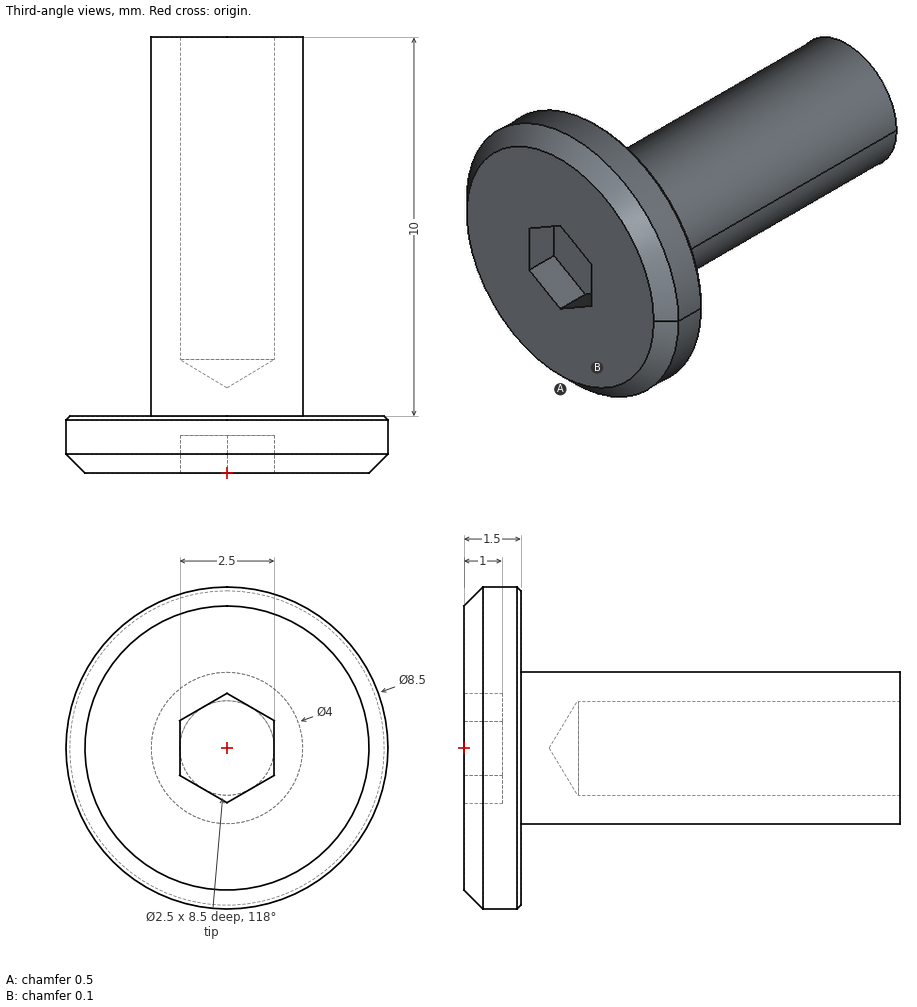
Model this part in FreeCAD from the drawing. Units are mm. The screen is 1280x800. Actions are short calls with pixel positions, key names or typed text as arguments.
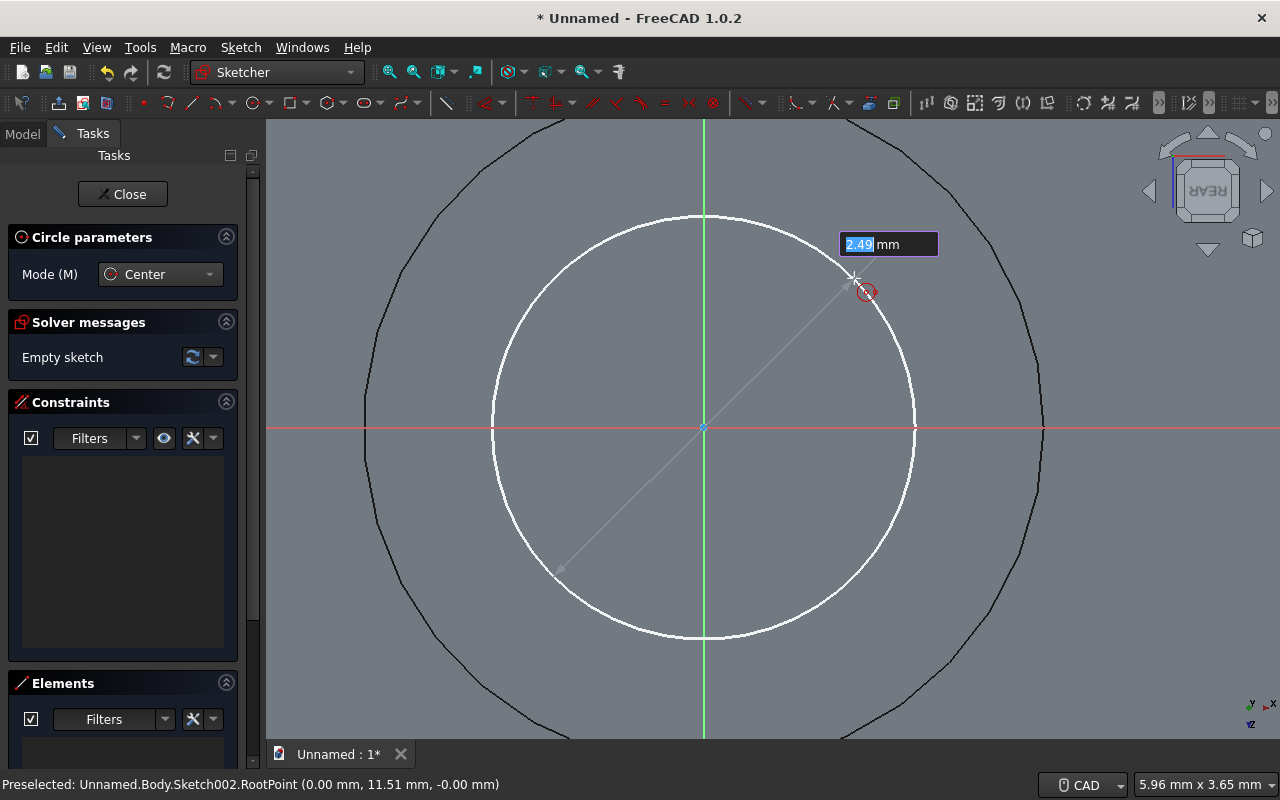
text(2.5)
key(Return)
key(Escape)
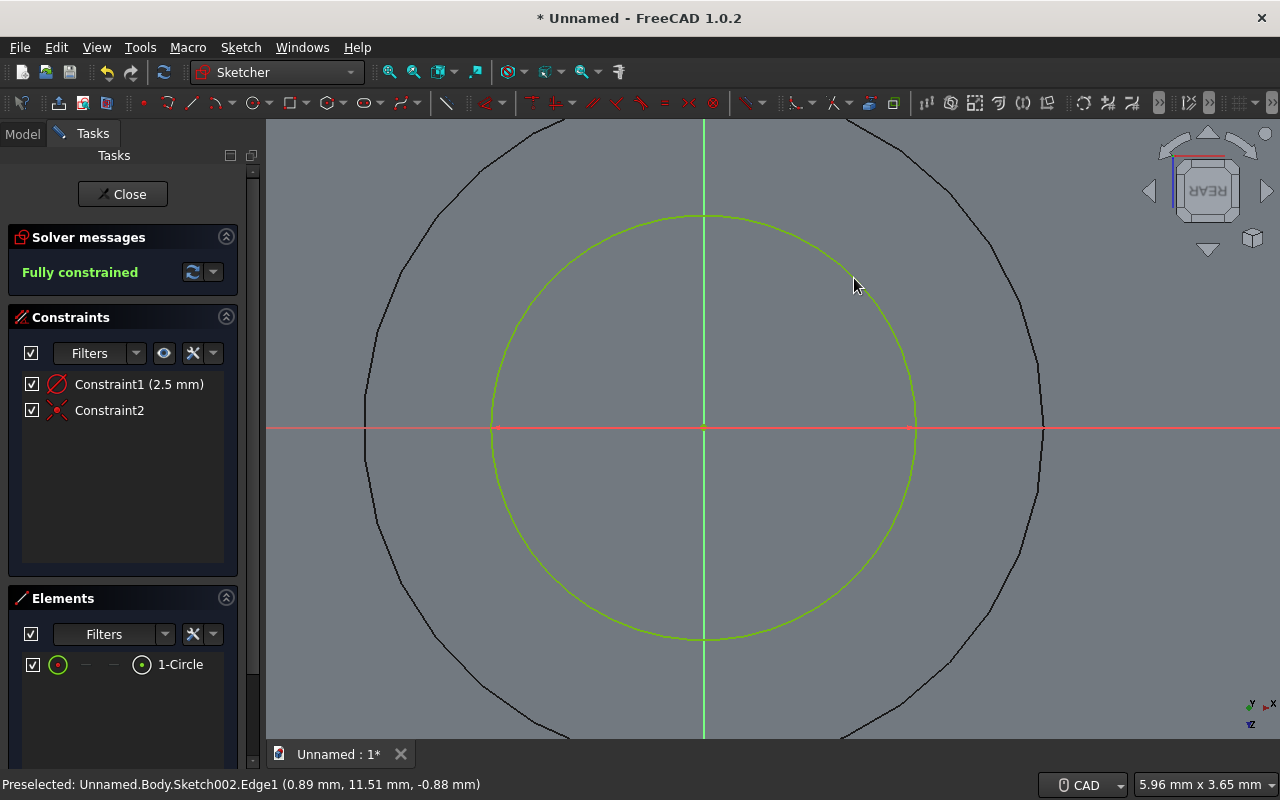
click(123, 194)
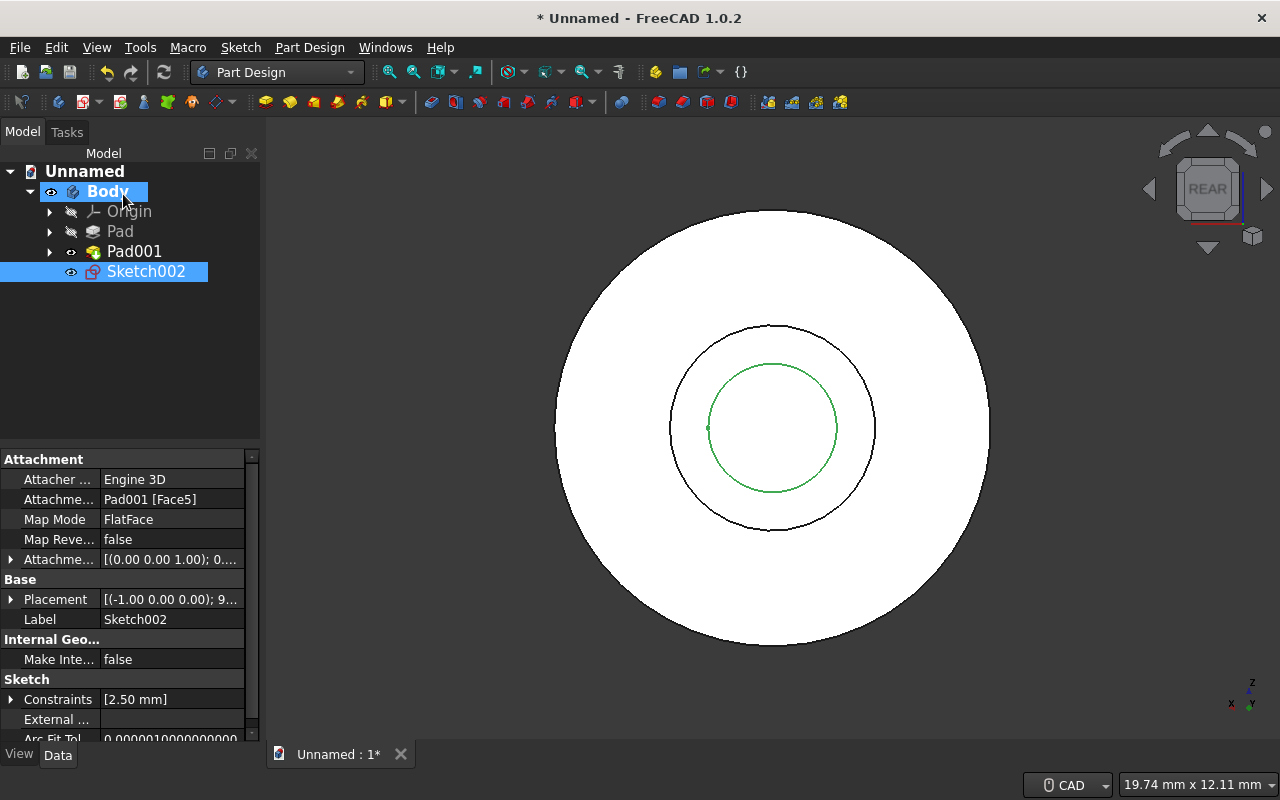
click(456, 102)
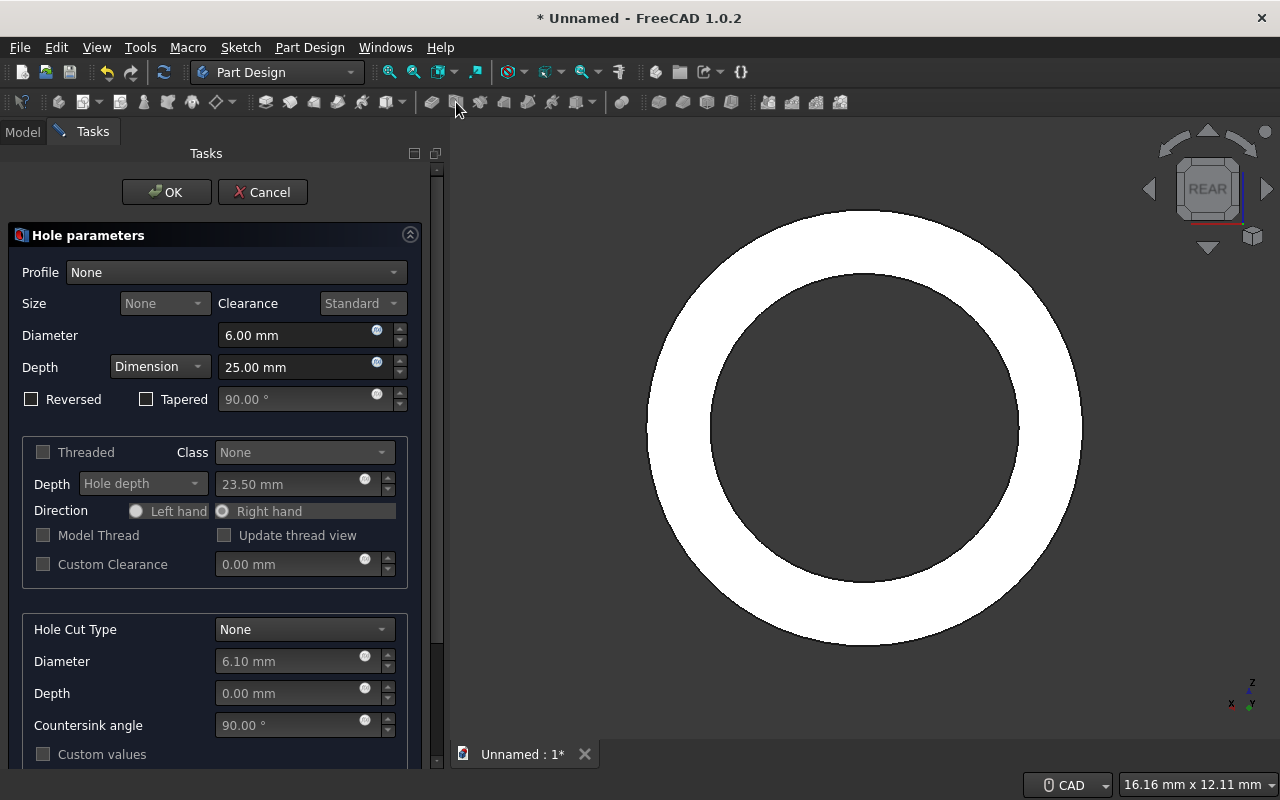
triple_click(305, 335)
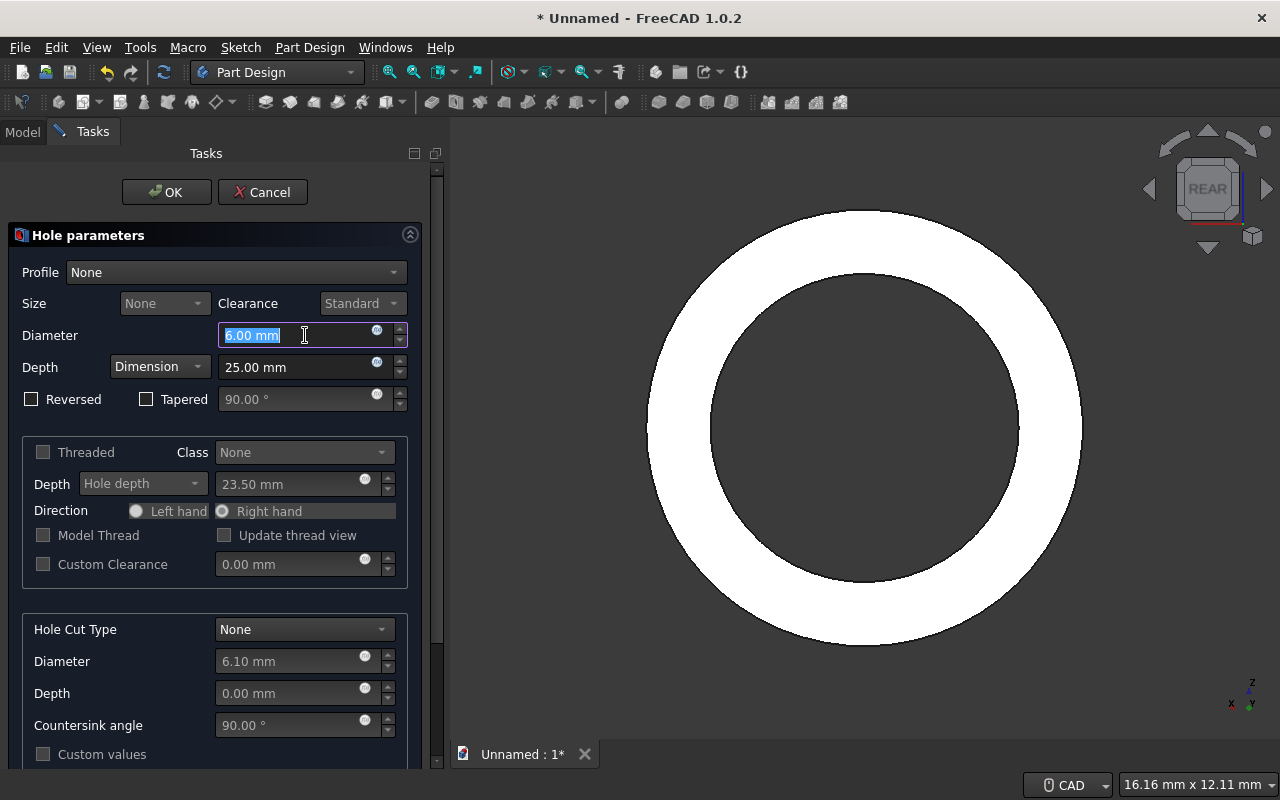
text(2.5)
key(Tab)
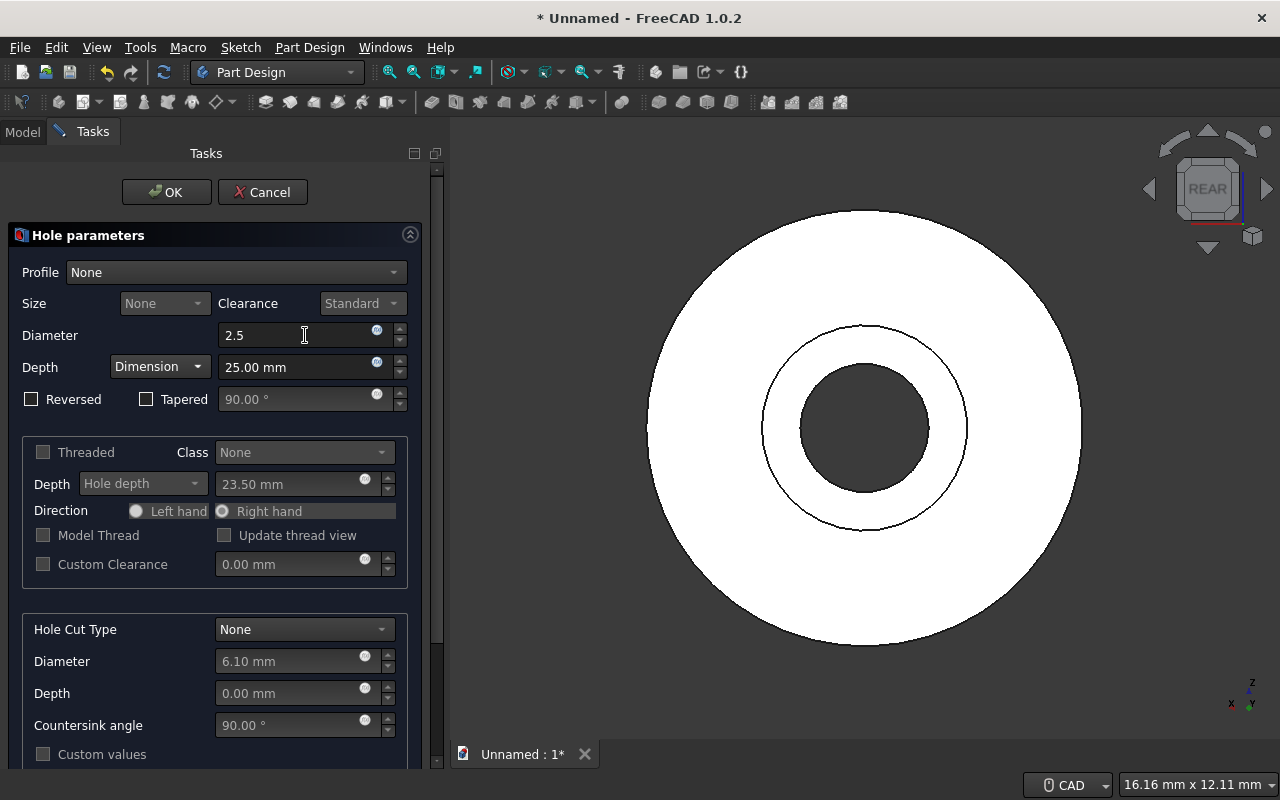
triple_click(305, 367)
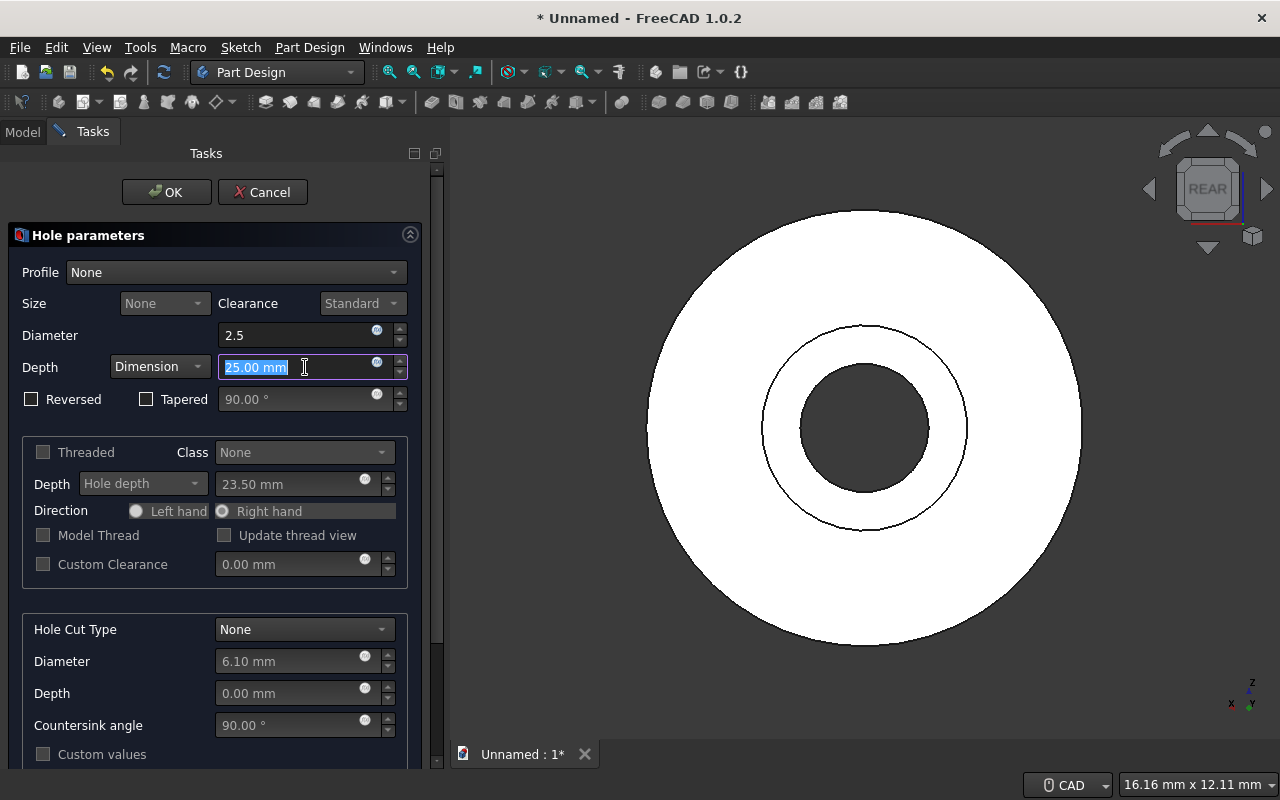
text(8.5)
key(Tab)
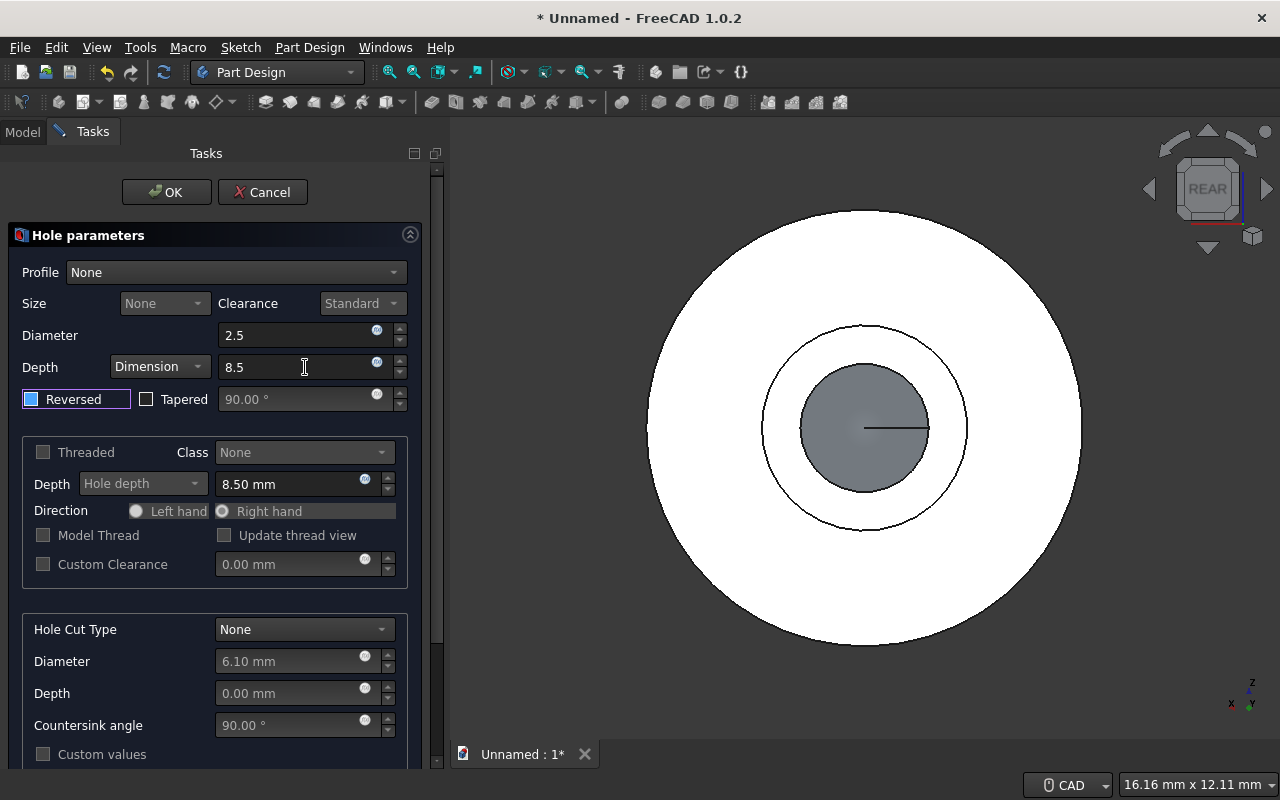
click(167, 192)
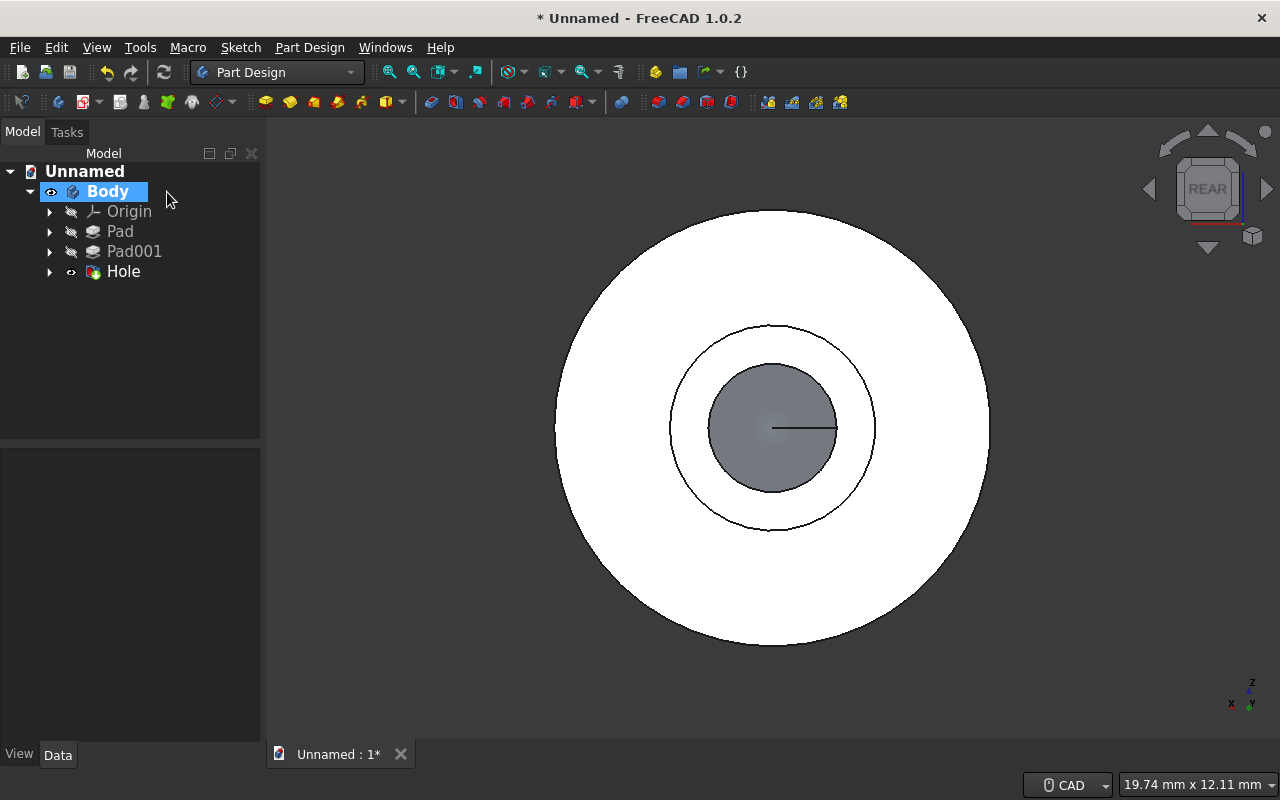
key(0)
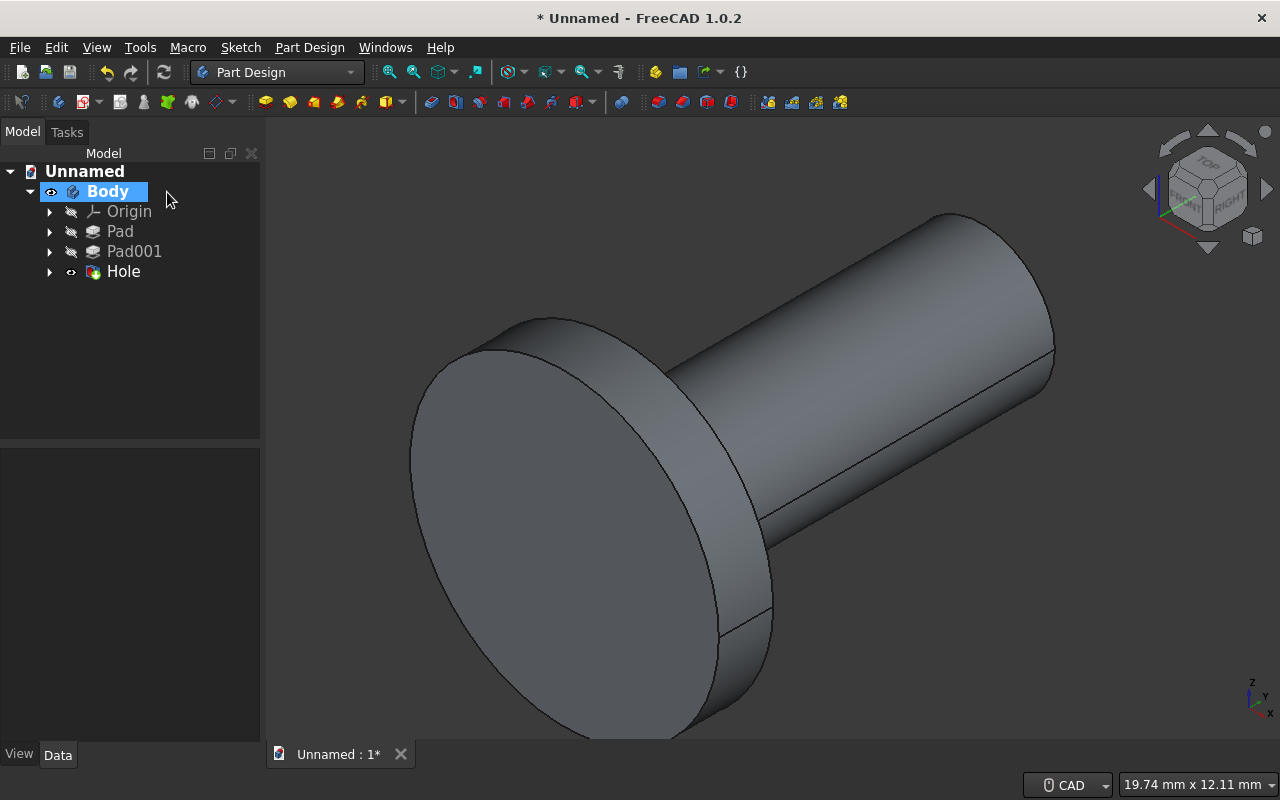
key(v)
key(f)